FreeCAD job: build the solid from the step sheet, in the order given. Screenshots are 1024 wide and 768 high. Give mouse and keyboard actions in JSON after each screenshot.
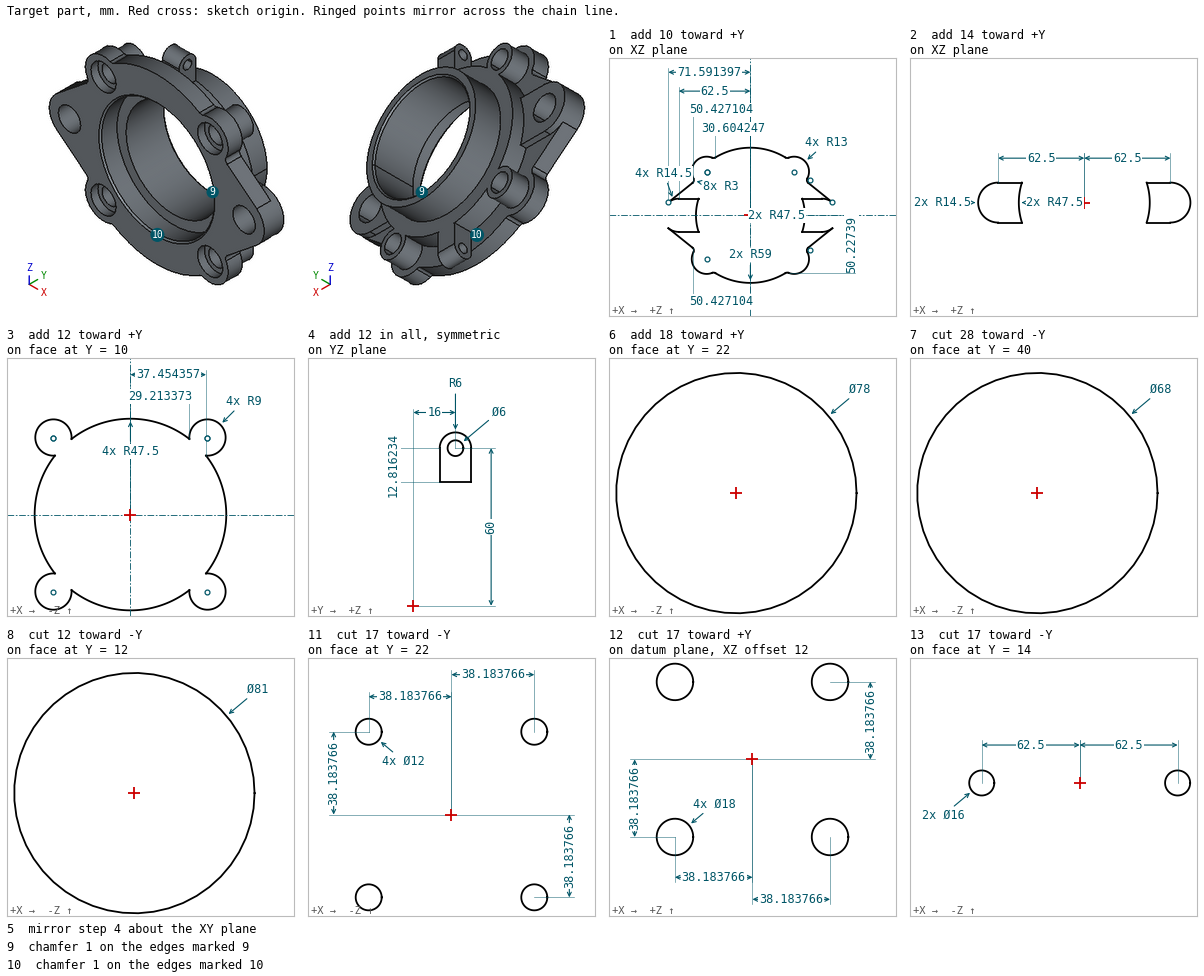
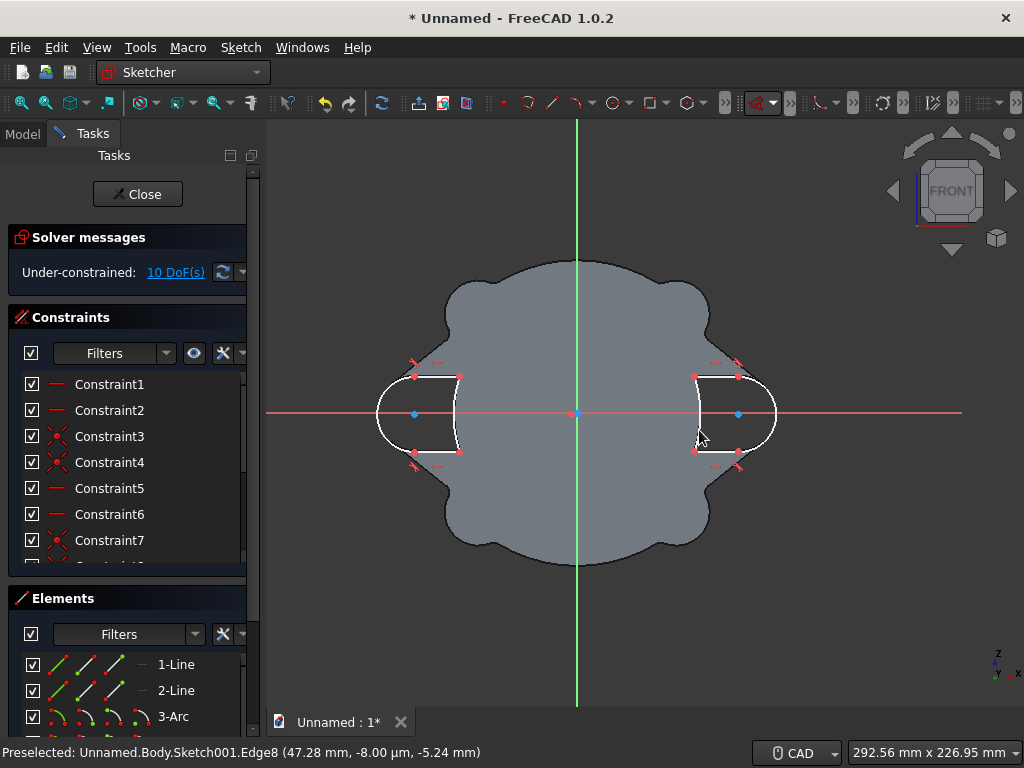
{"action": "left_click_drag", "start_coordinate": [561, 403], "coordinate": [587, 425]}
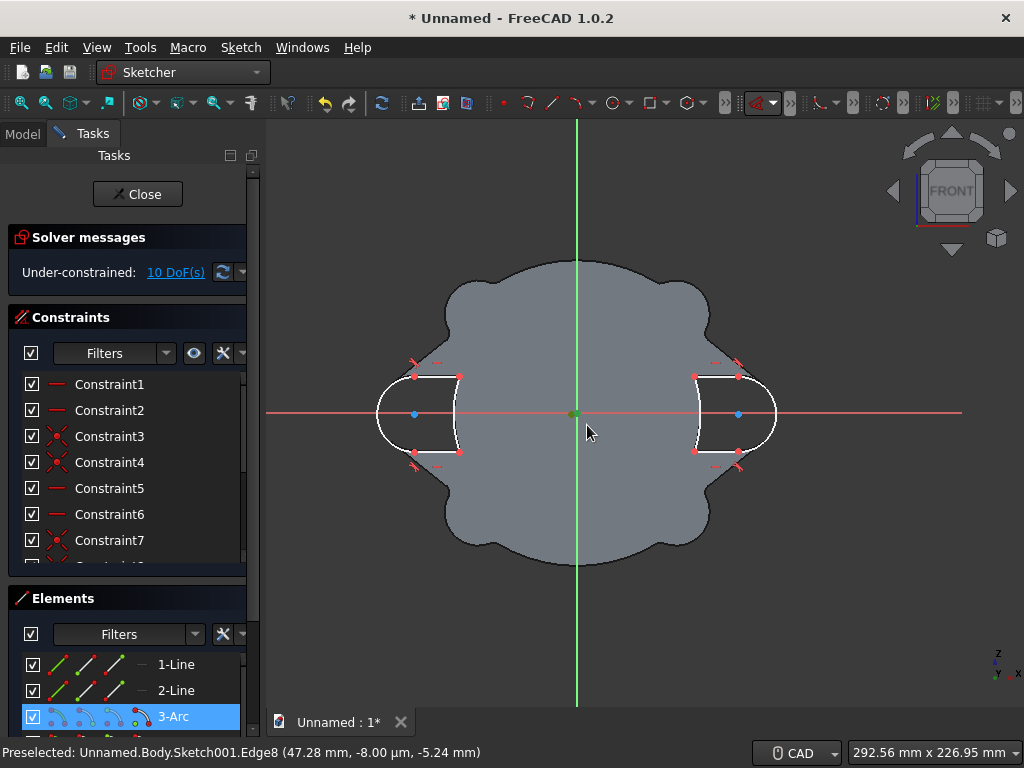
{"action": "key", "text": "c"}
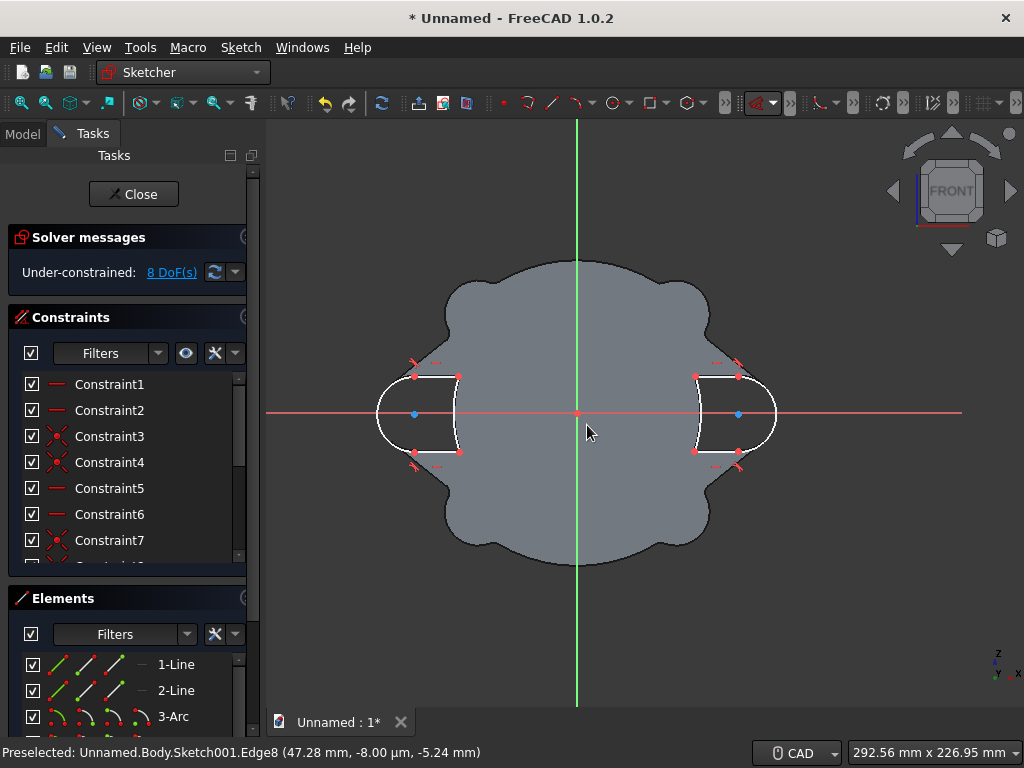
{"action": "left_click", "coordinate": [384, 392]}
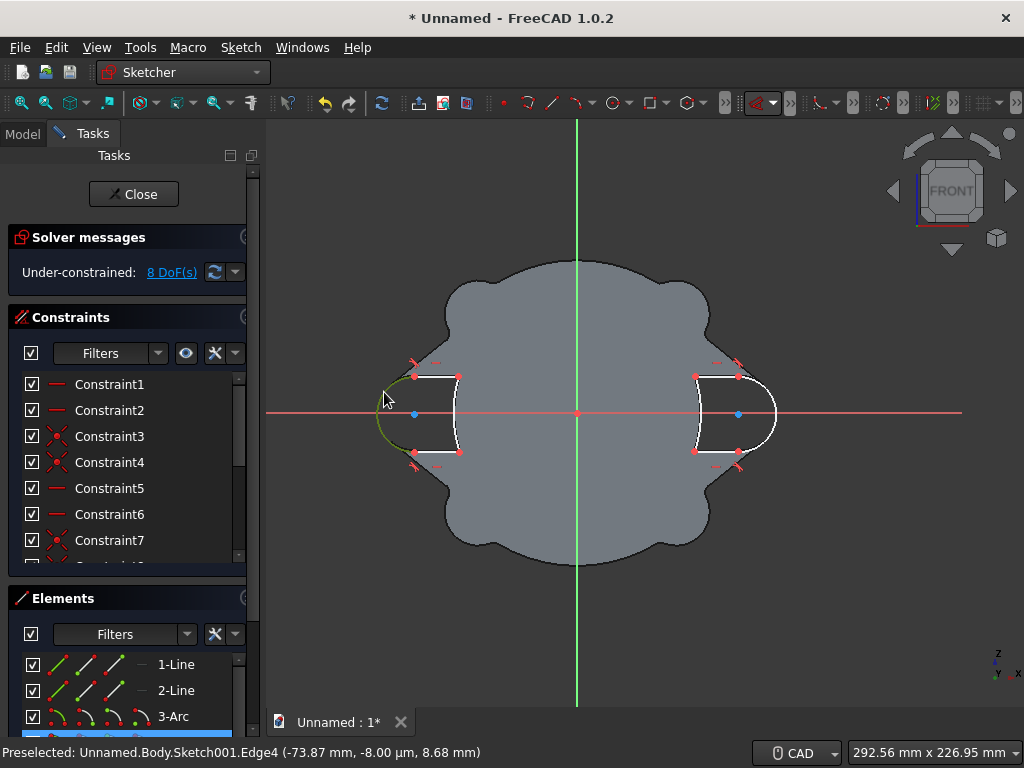
{"action": "left_click", "coordinate": [769, 437]}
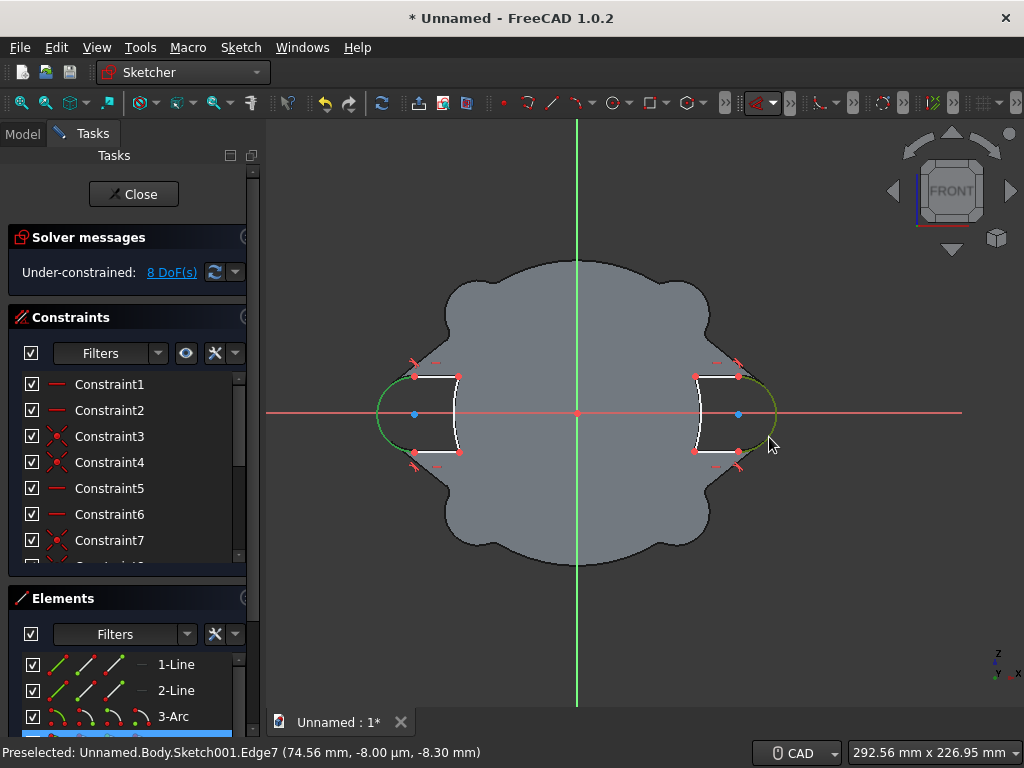
{"action": "key", "text": "e"}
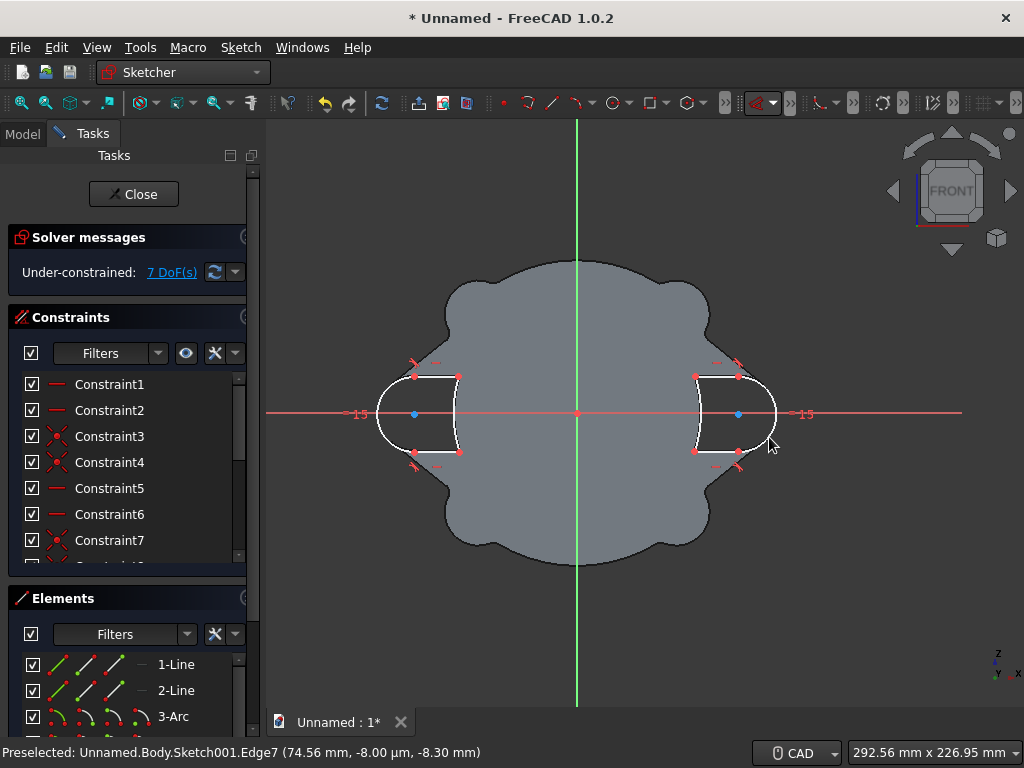
{"action": "left_click", "coordinate": [454, 399]}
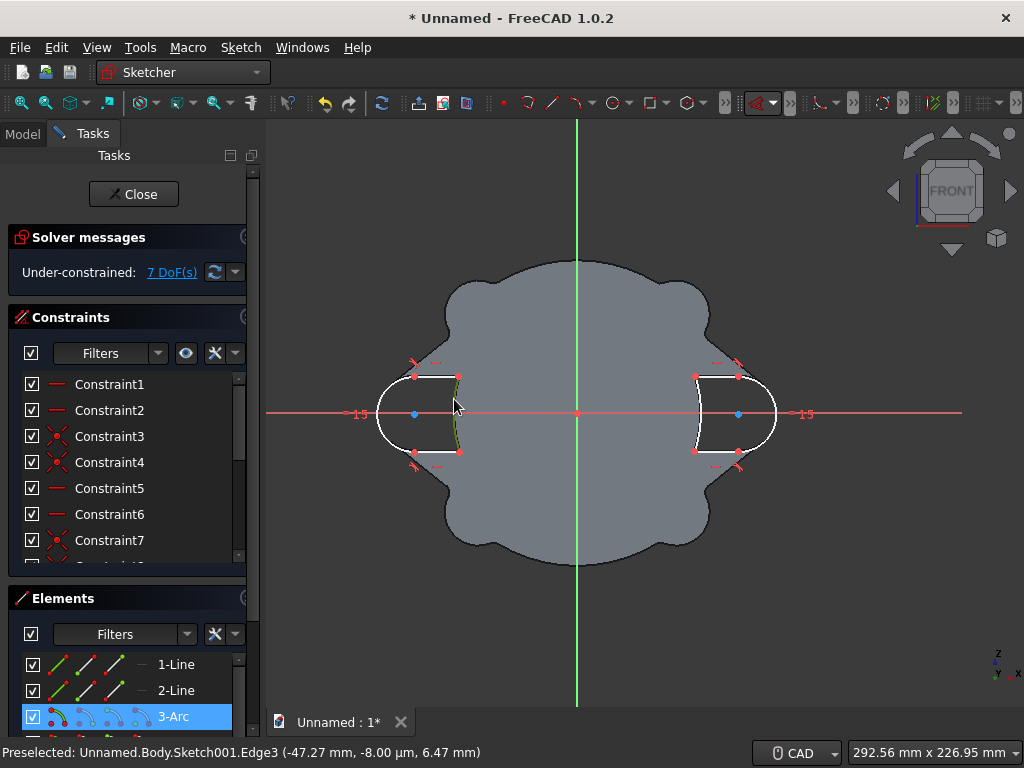
{"action": "left_click", "coordinate": [700, 430]}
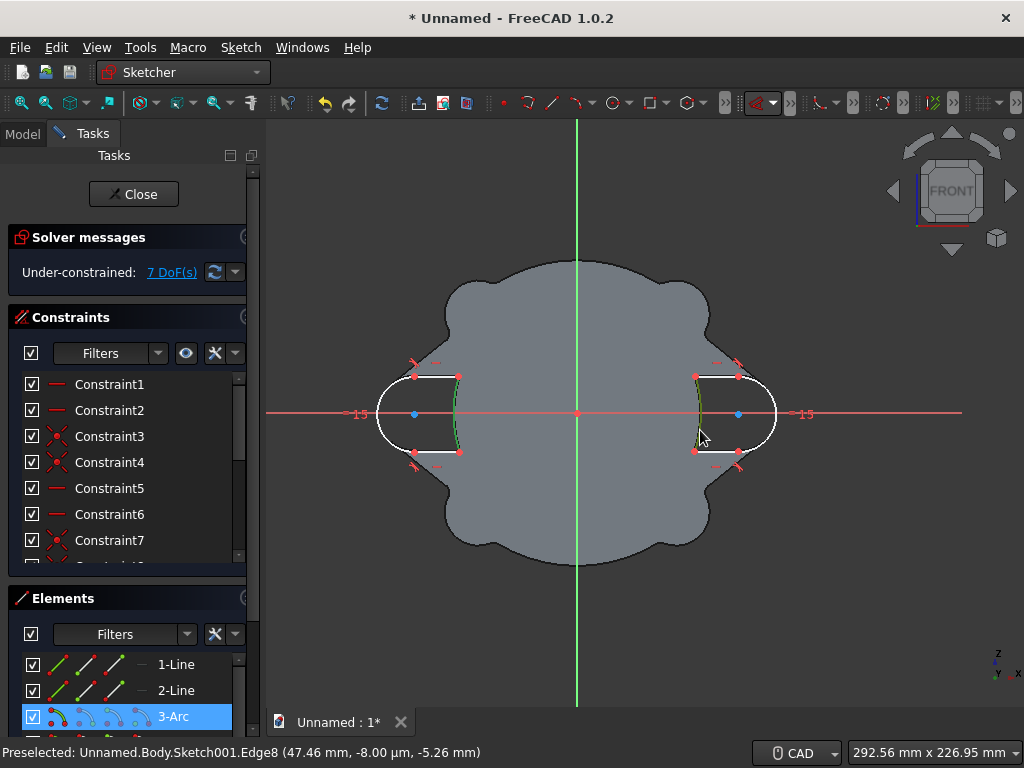
{"action": "key", "text": "e"}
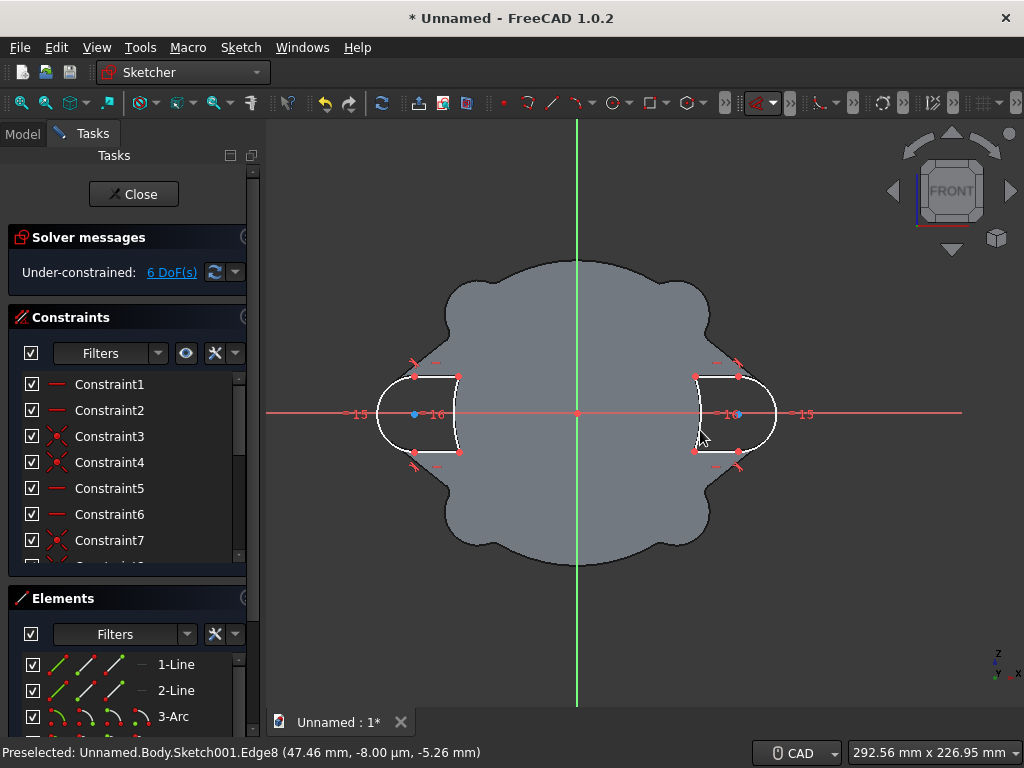
{"action": "left_click", "coordinate": [415, 414]}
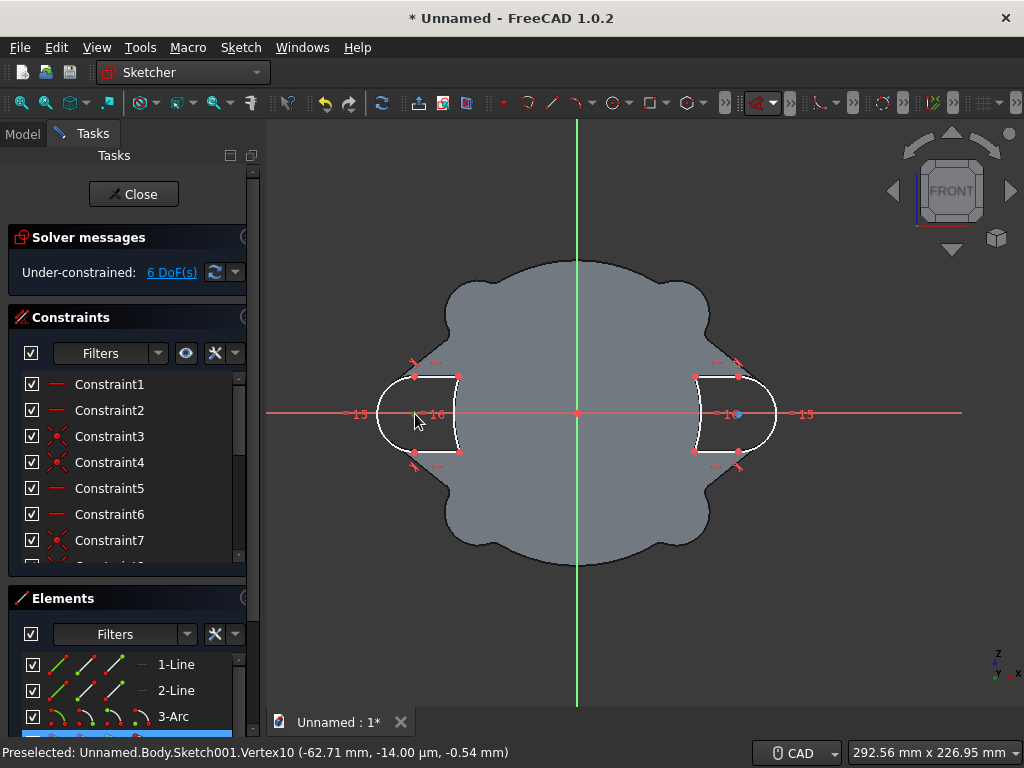
{"action": "left_click", "coordinate": [334, 413]}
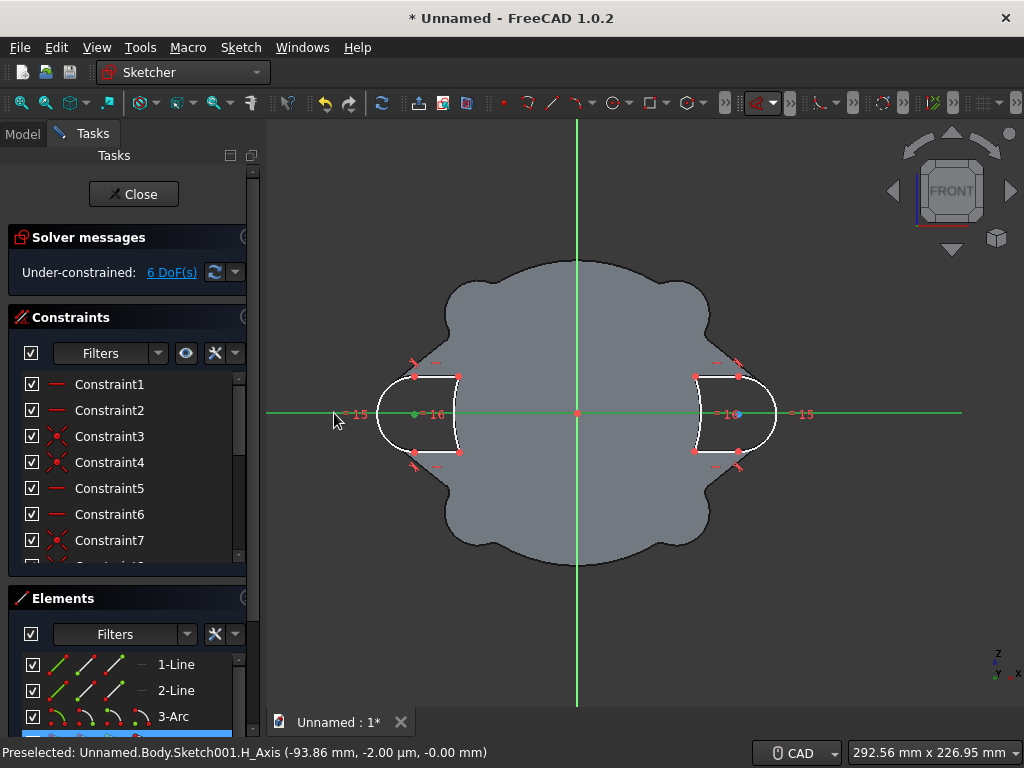
{"action": "key", "text": "c"}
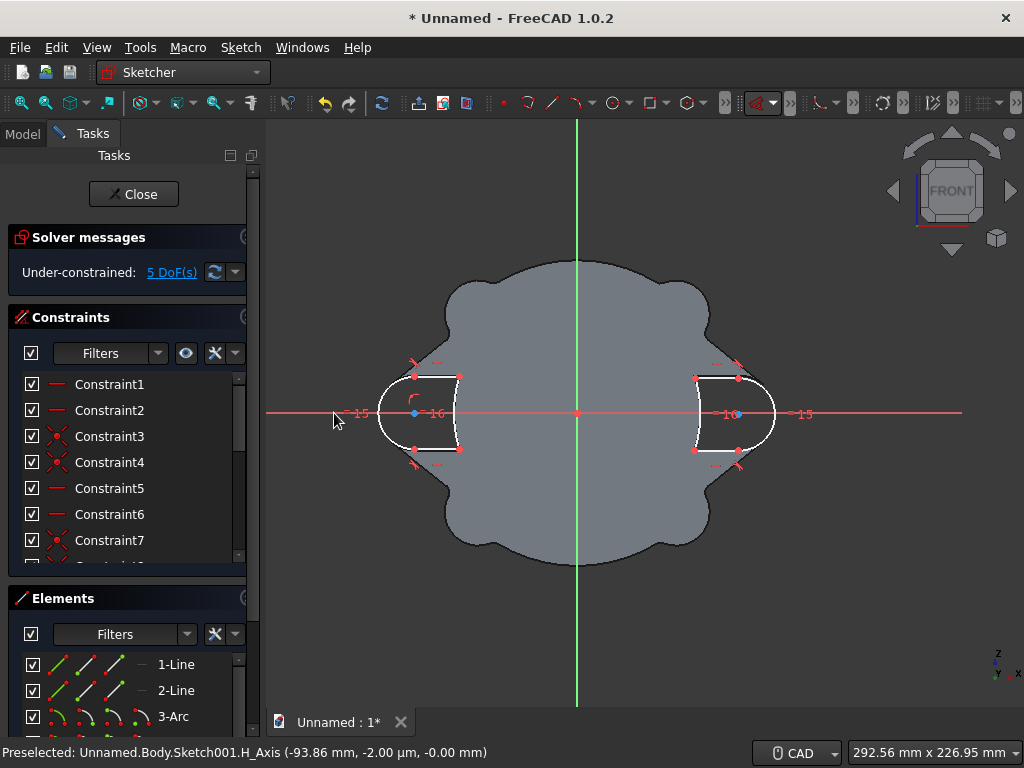
{"action": "left_click", "coordinate": [739, 414]}